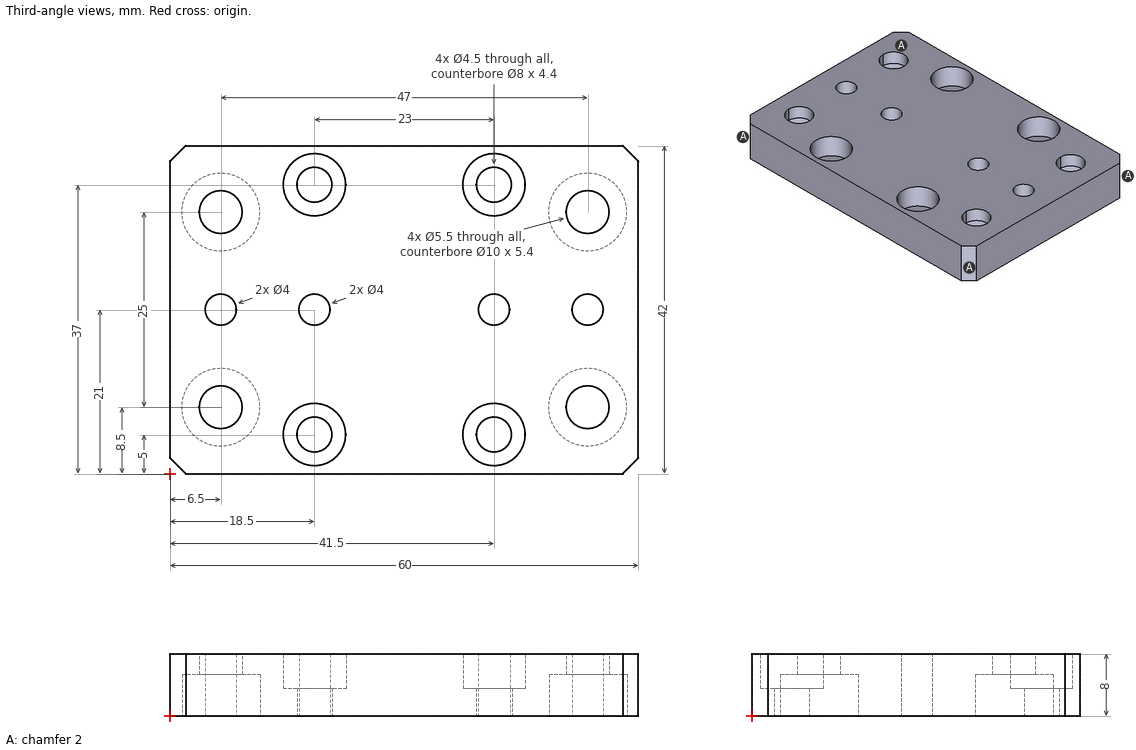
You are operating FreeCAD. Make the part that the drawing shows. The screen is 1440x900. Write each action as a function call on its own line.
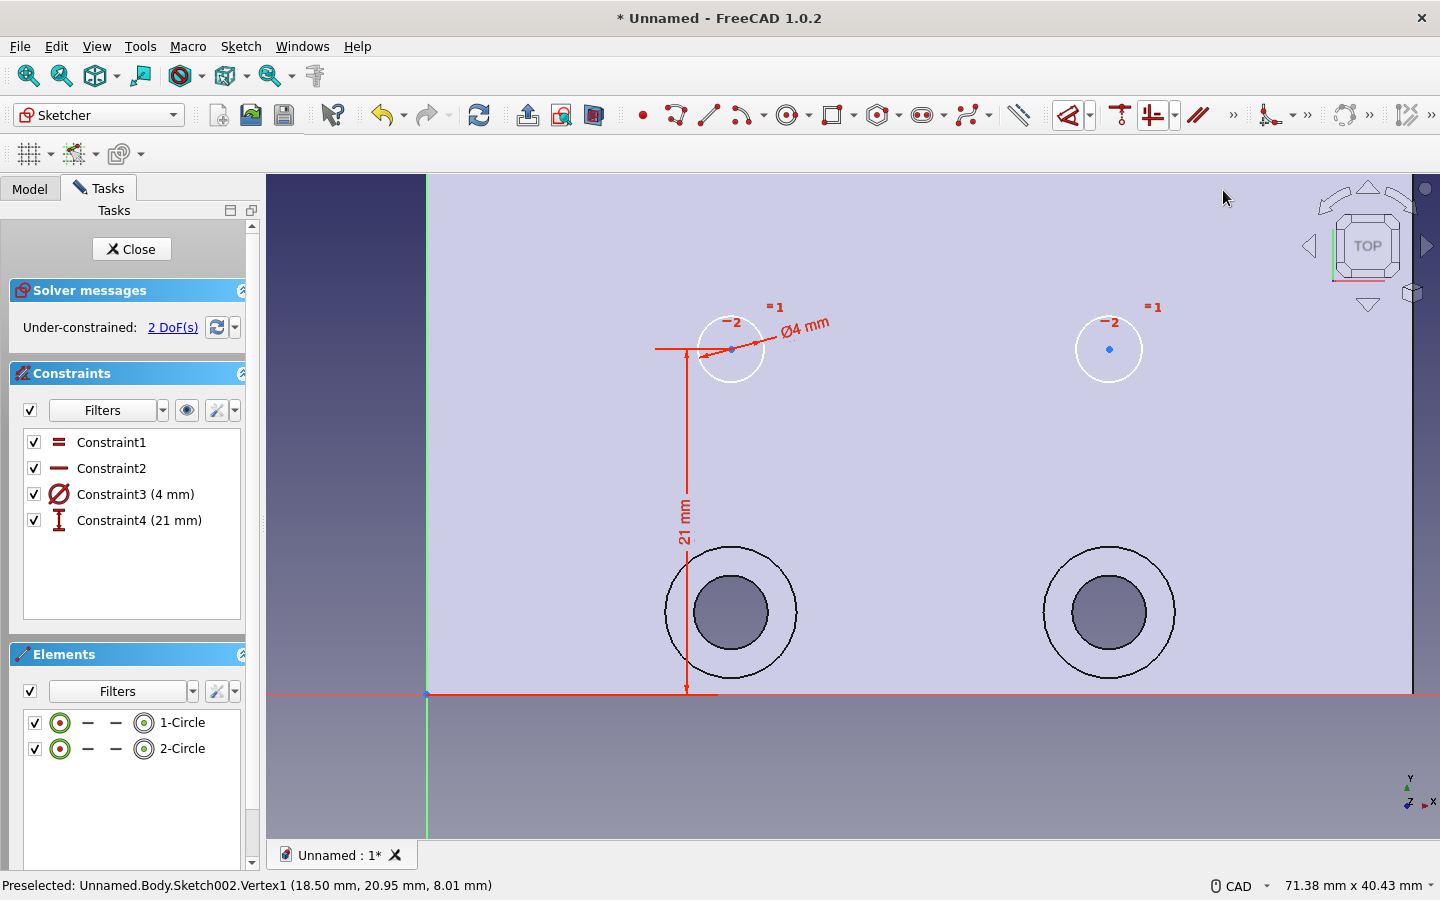
click(731, 349)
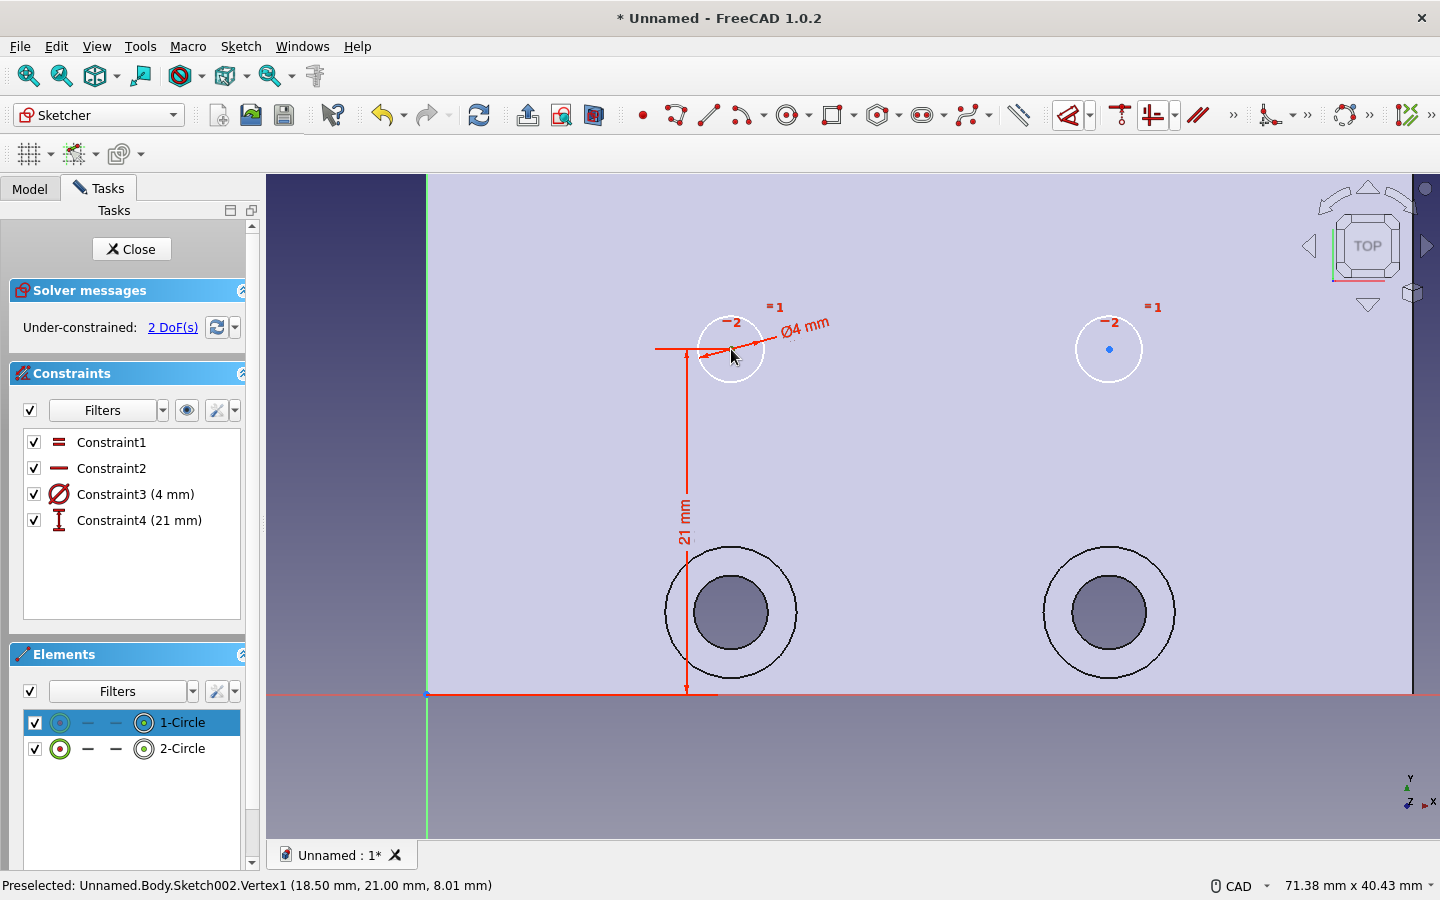
click(1109, 349)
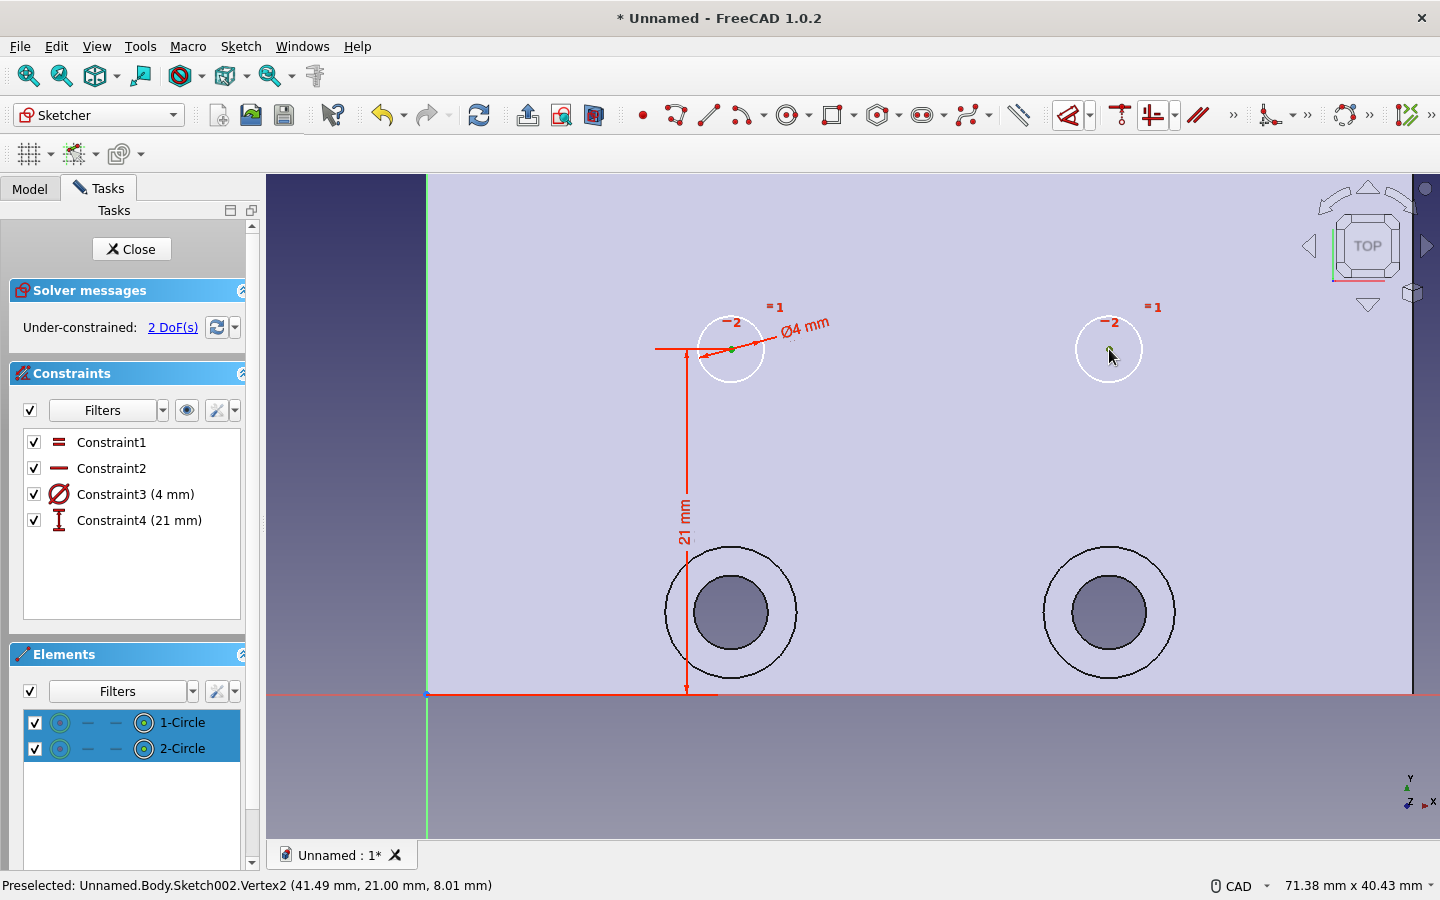
key(l)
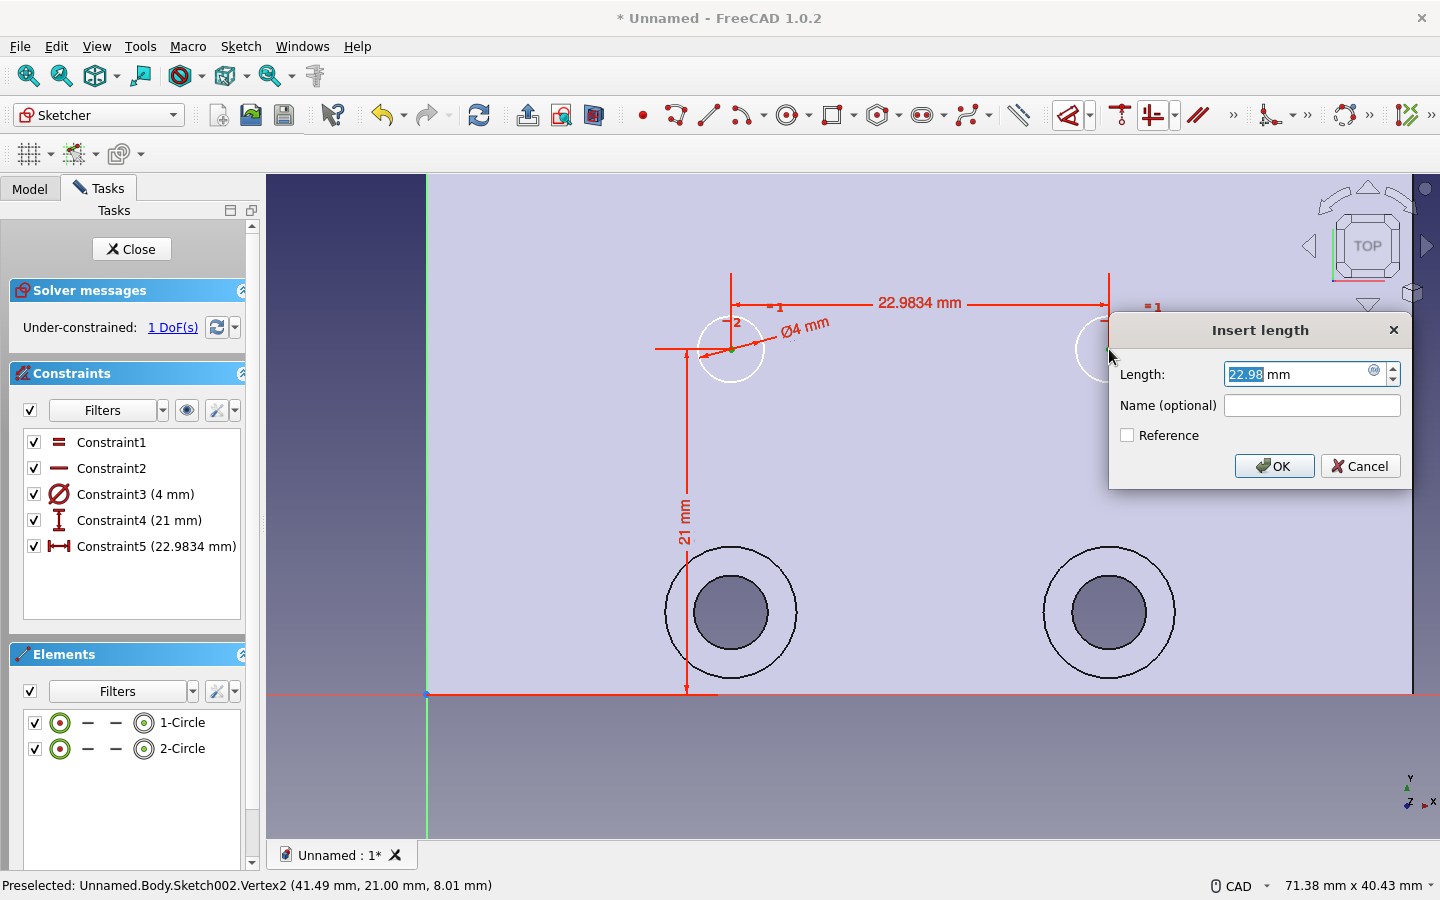
text(23)
key(Return)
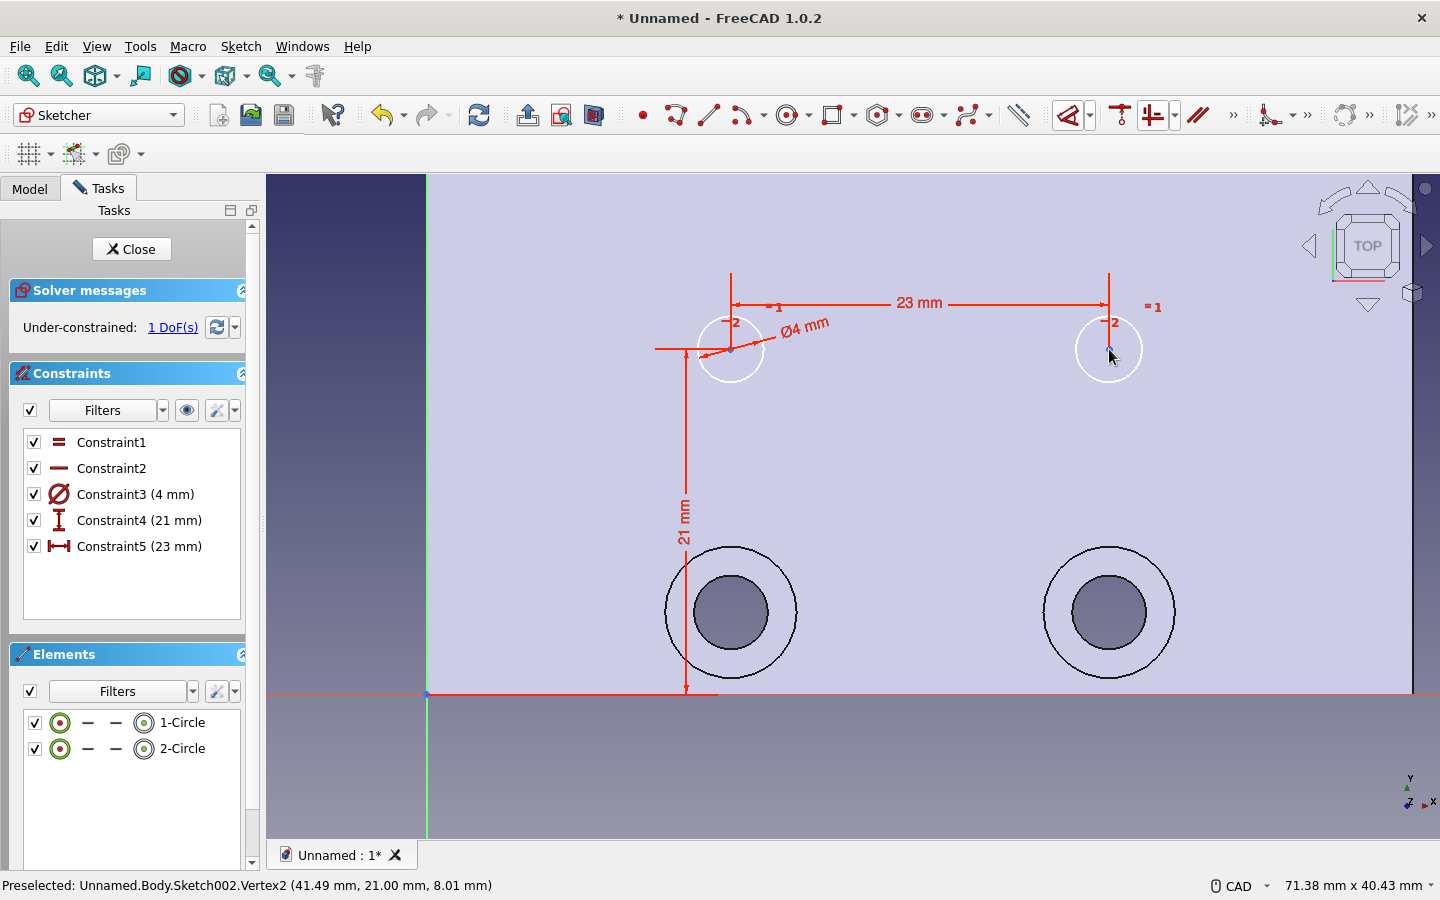
click(731, 349)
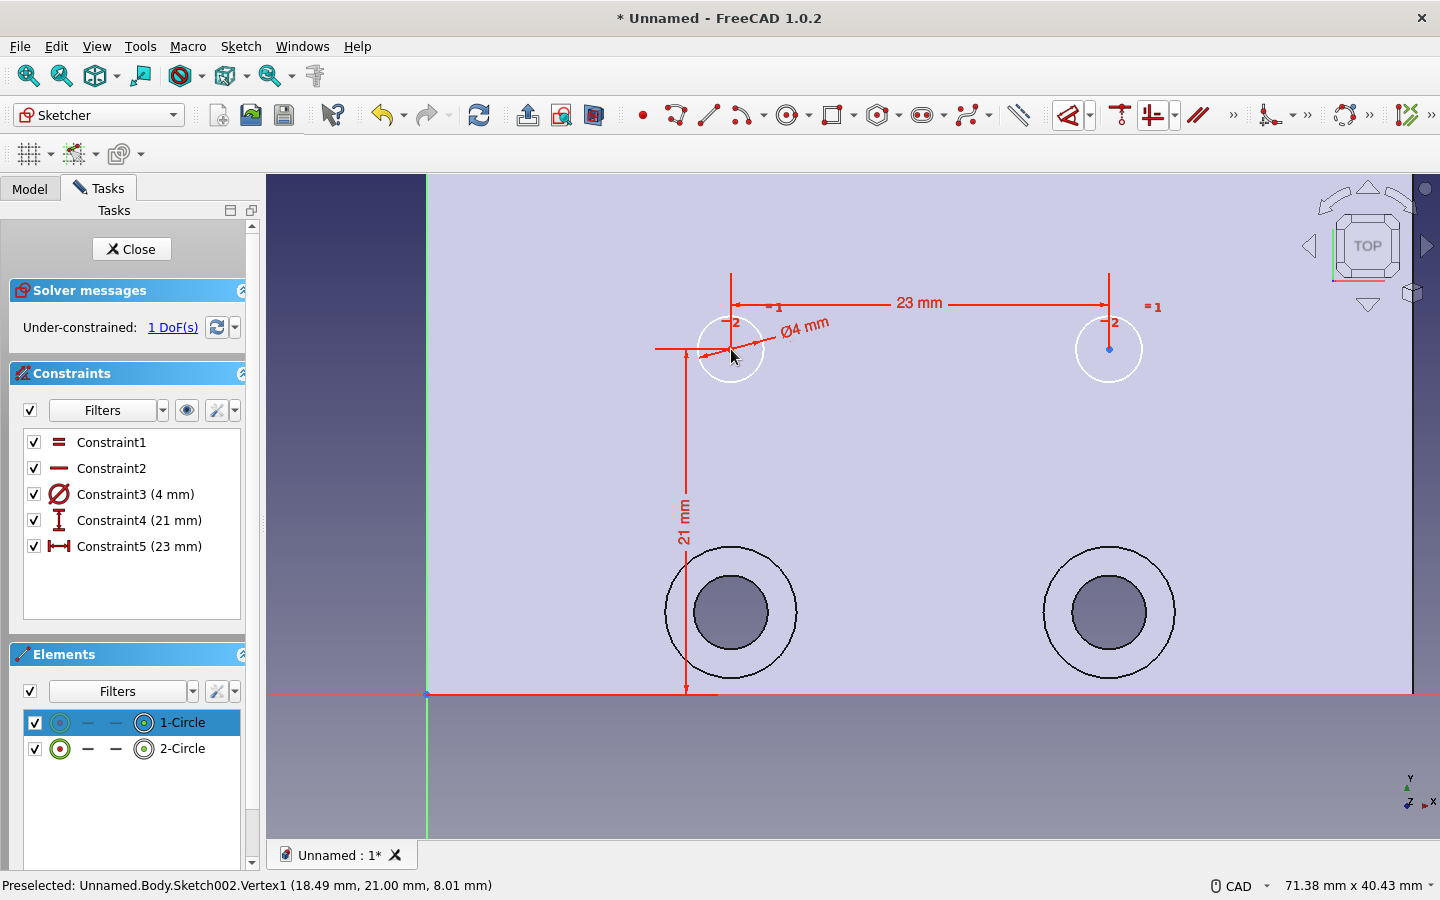
key(l)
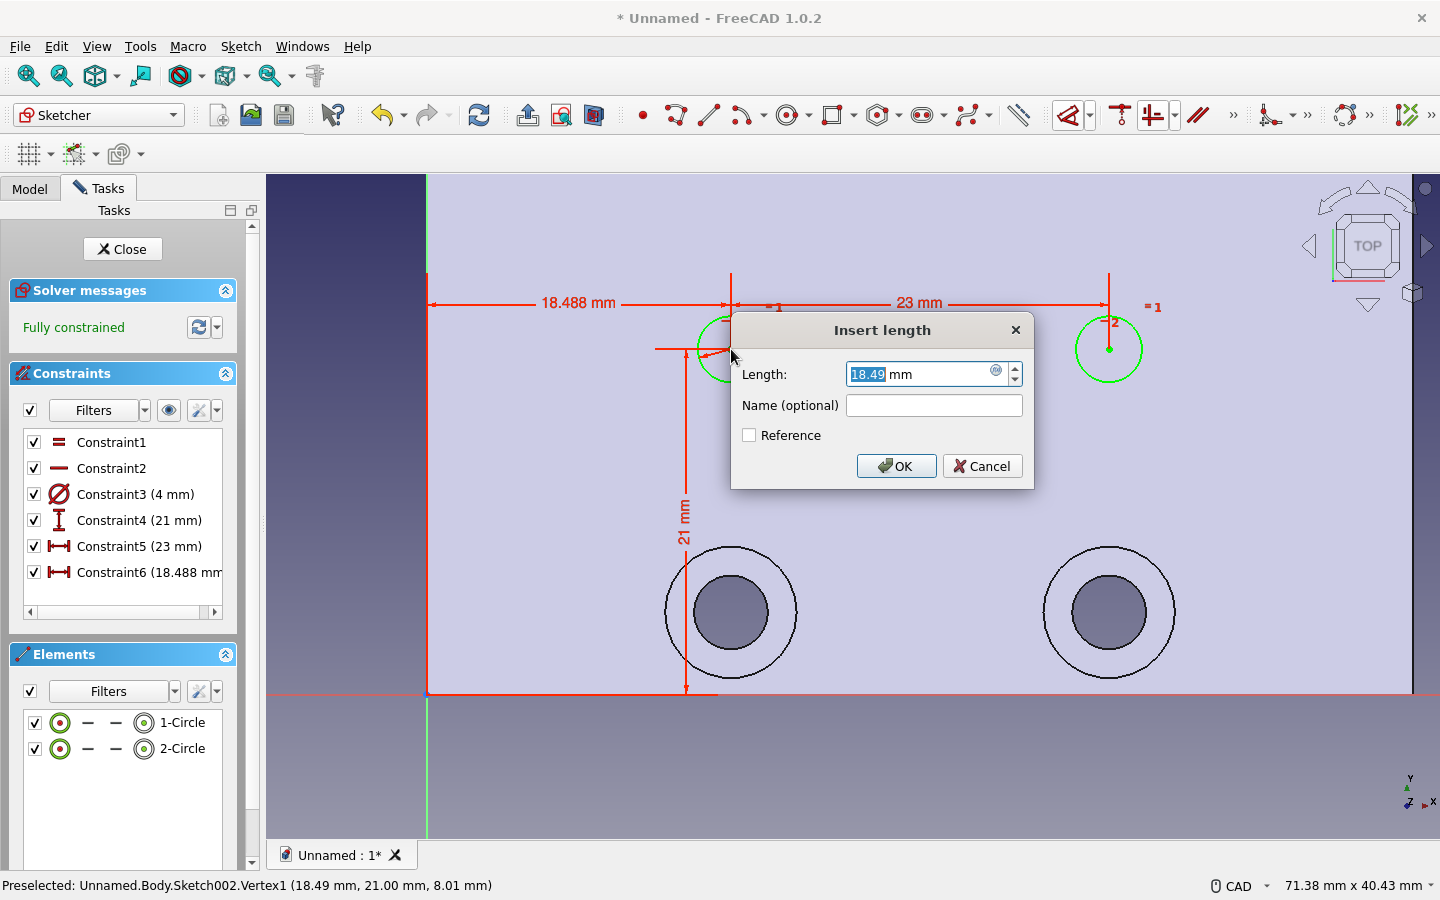
text(18.5)
key(Return)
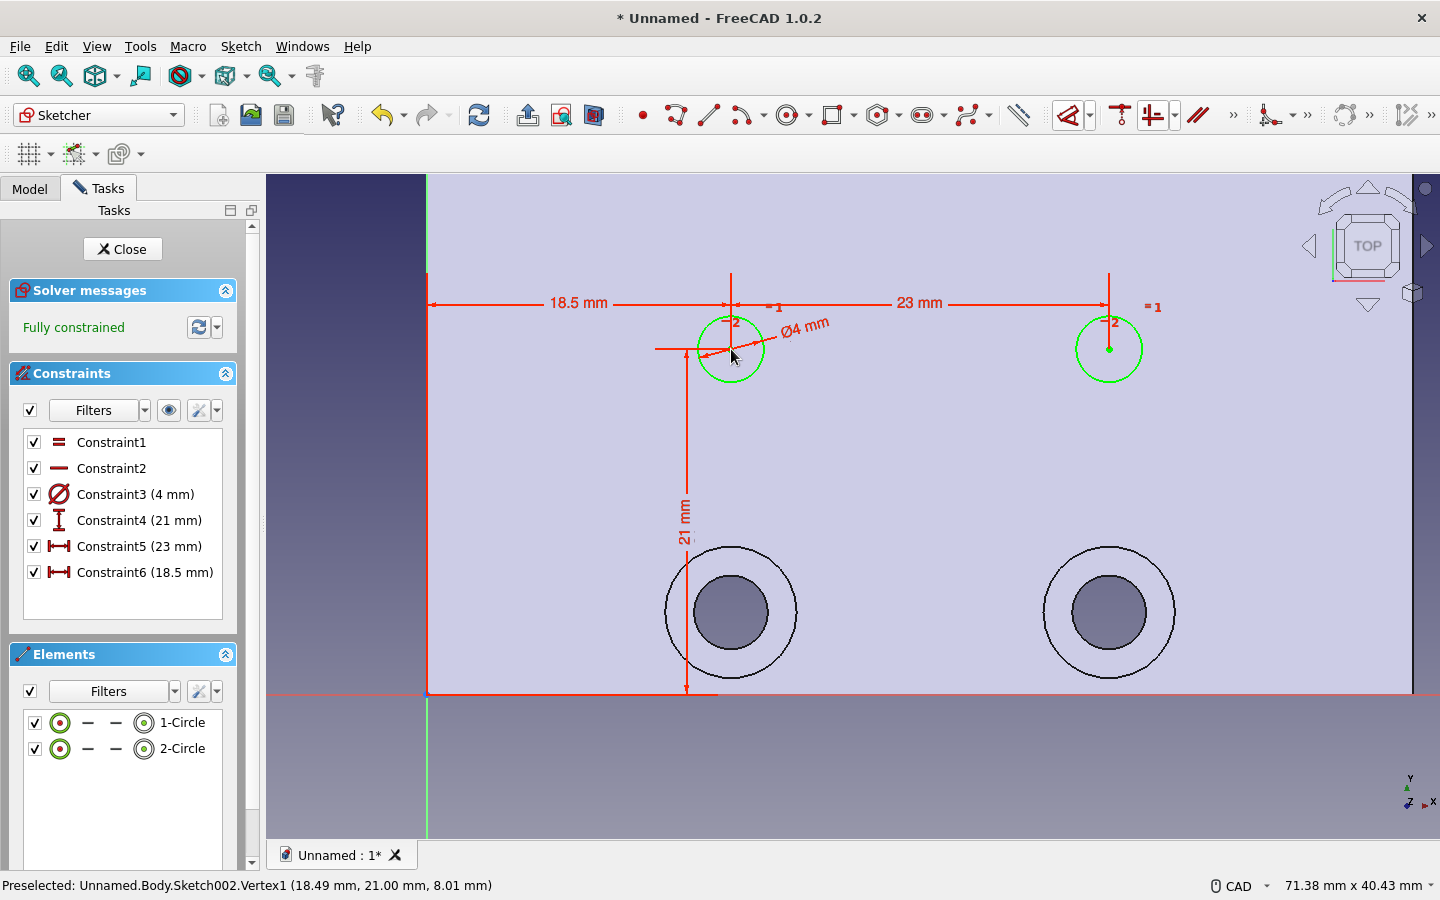
click(123, 249)